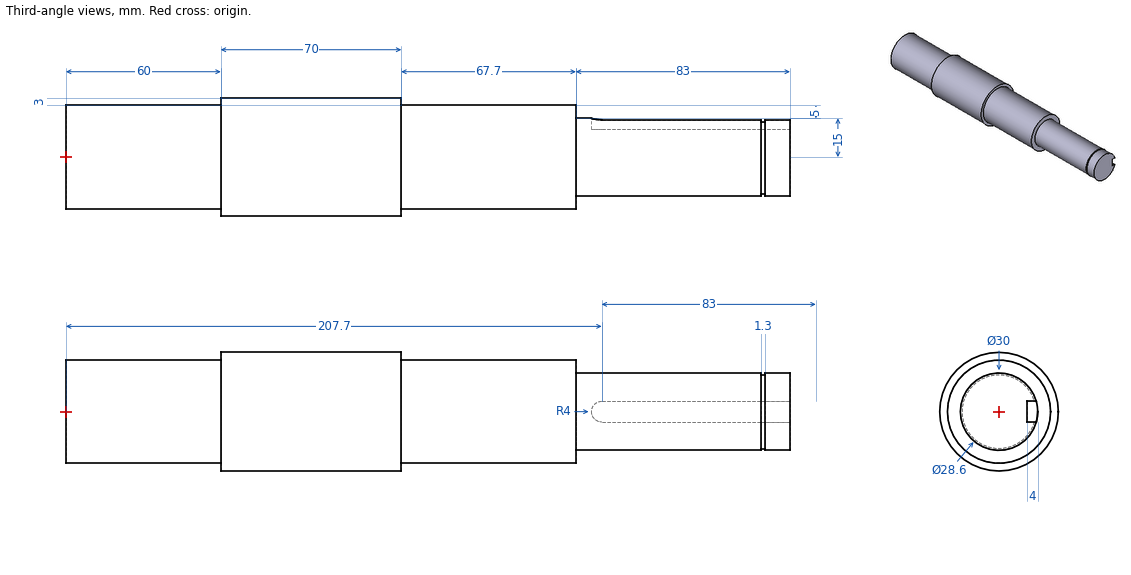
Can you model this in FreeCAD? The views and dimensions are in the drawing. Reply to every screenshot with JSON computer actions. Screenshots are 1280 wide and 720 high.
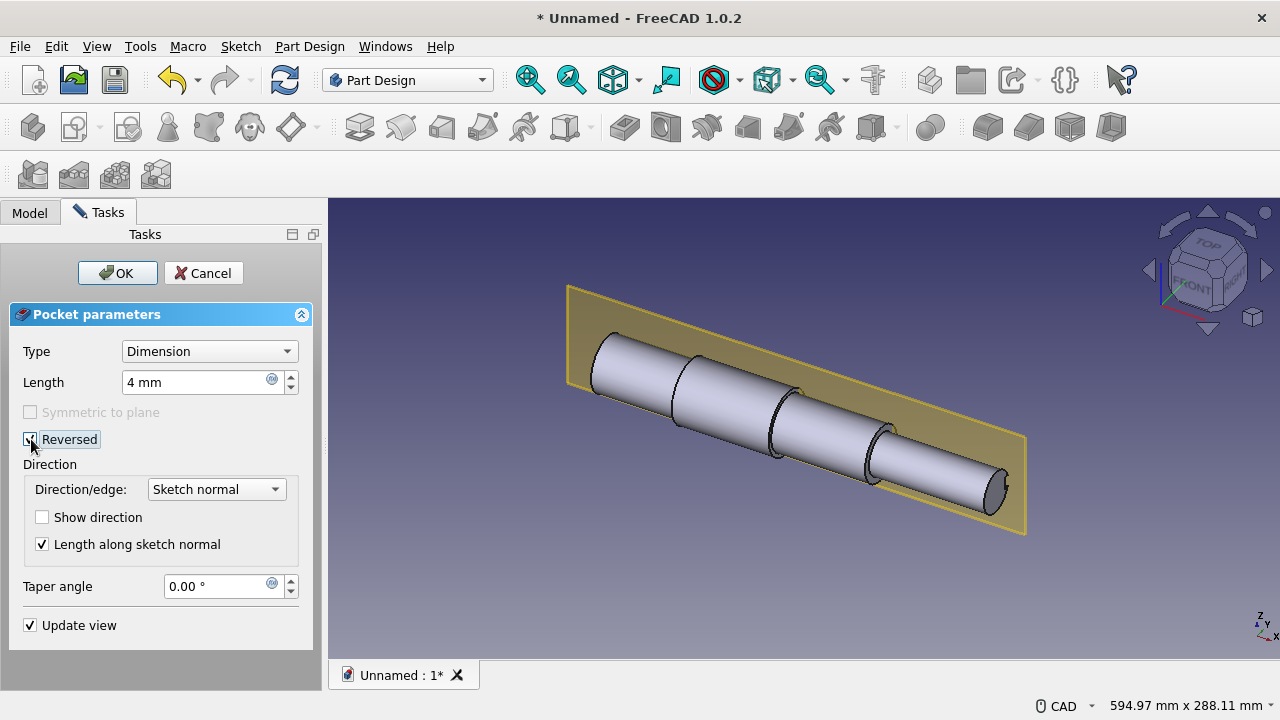
{"action": "left_click", "coordinate": [118, 273]}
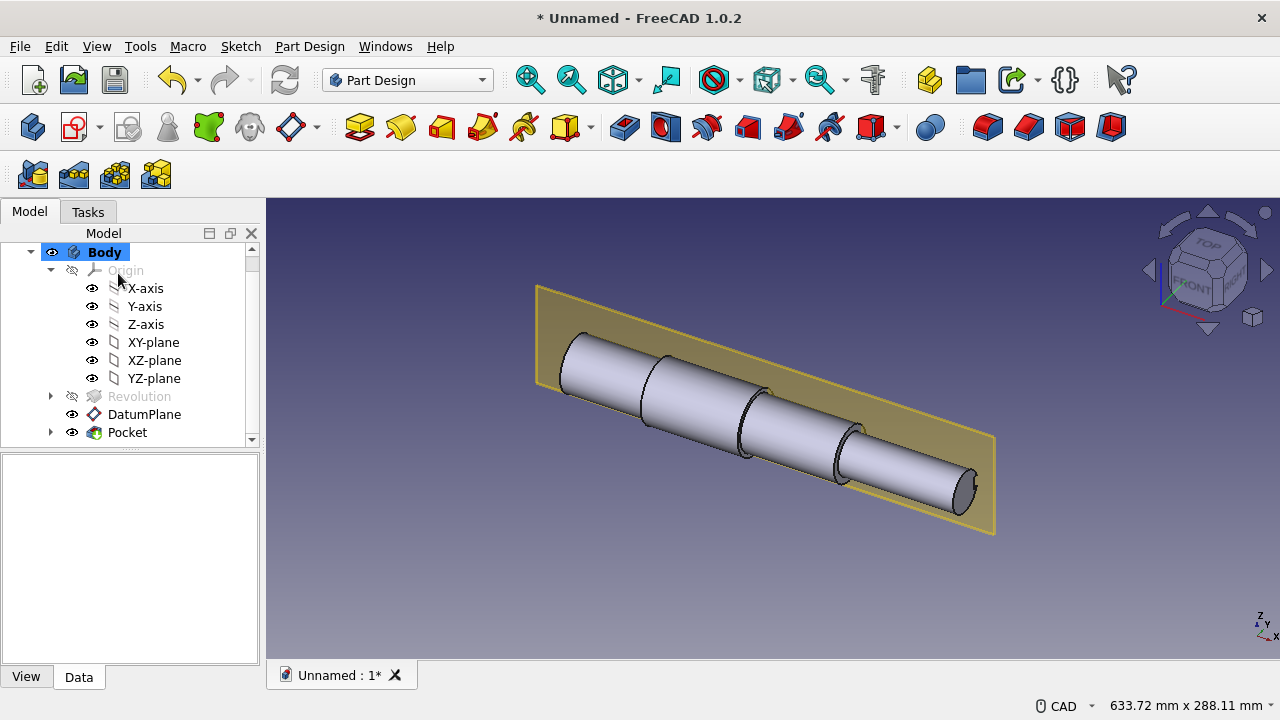
{"action": "left_click", "coordinate": [117, 414]}
{"action": "key", "text": "space"}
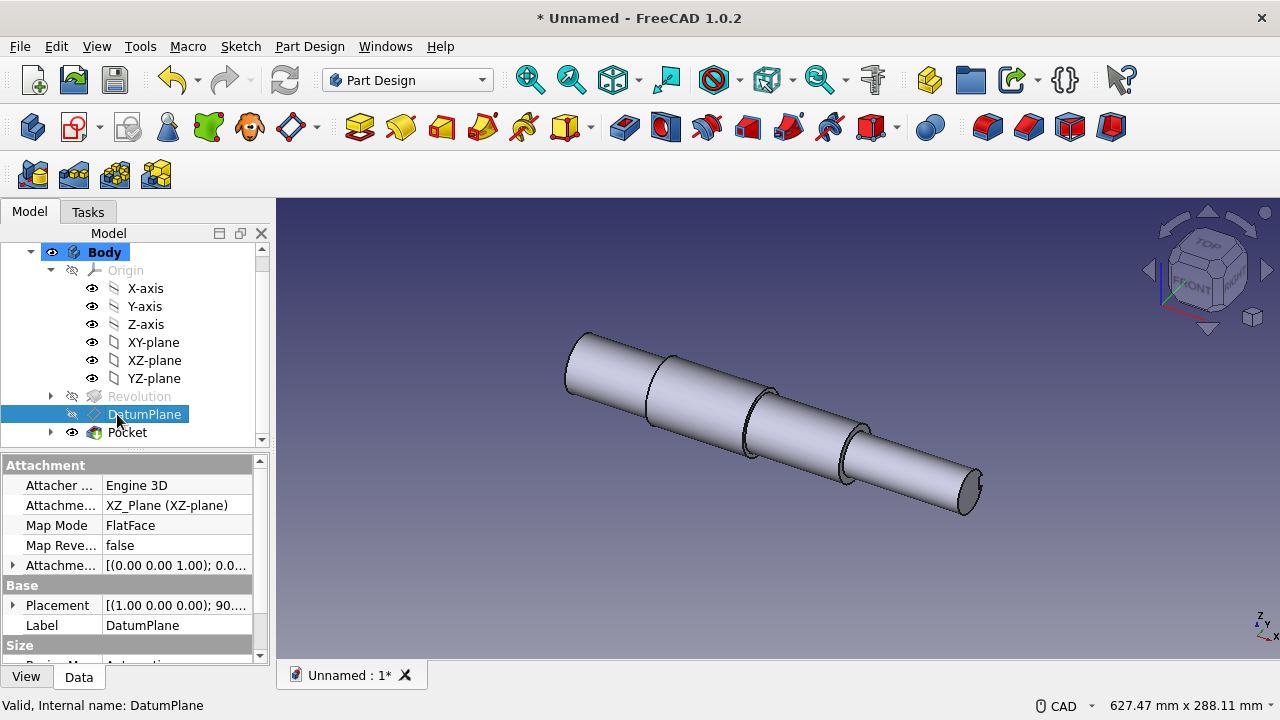
{"action": "left_click", "coordinate": [137, 378]}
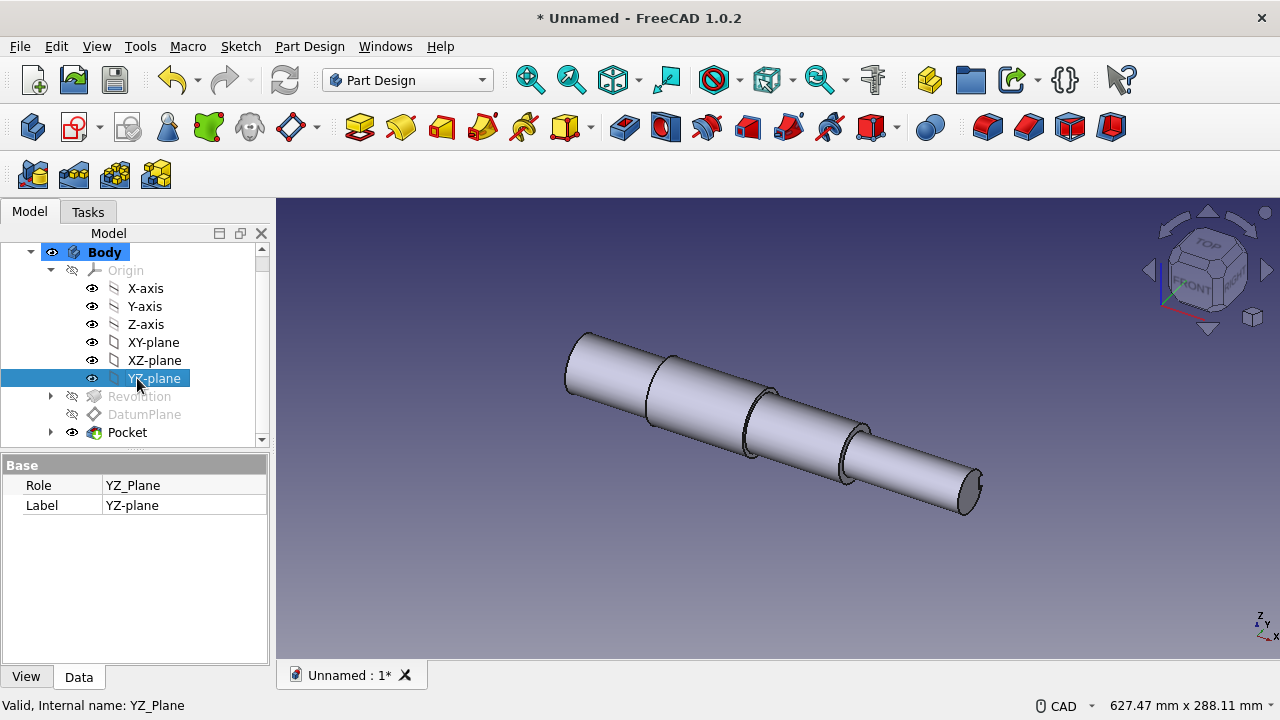
{"action": "left_click", "coordinate": [290, 128]}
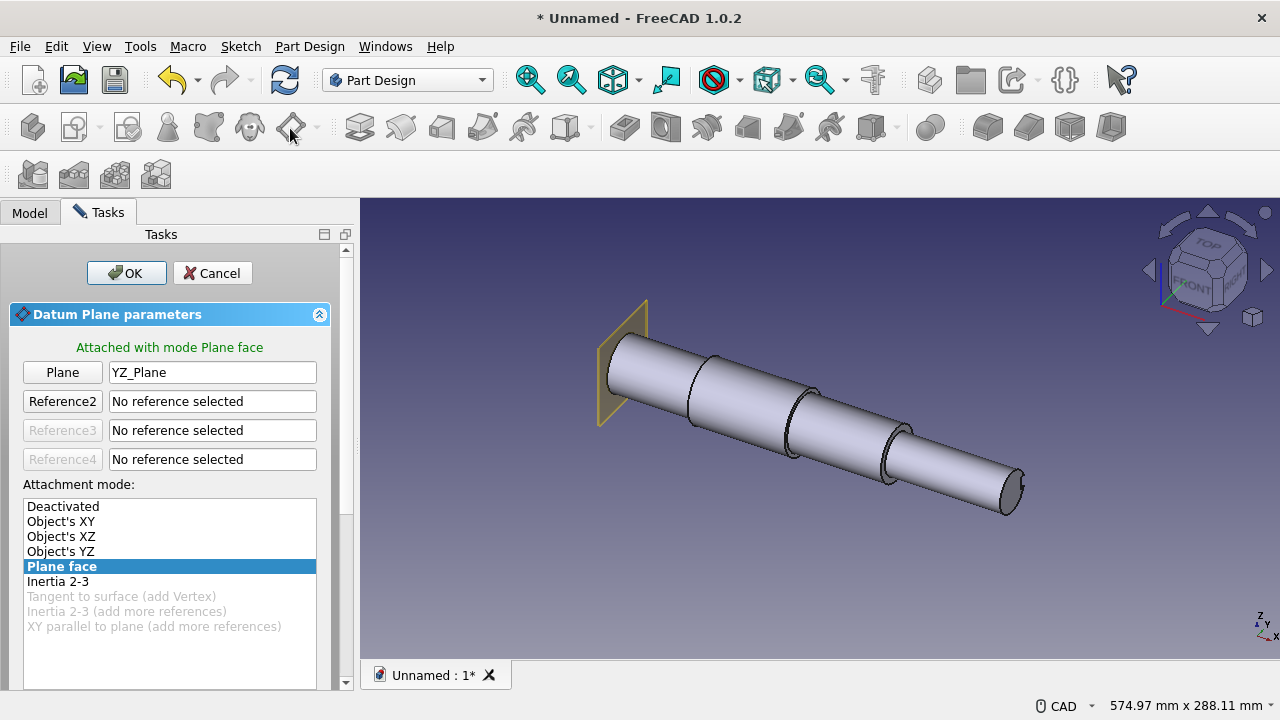
{"action": "scroll", "coordinate": [346, 467], "scroll_direction": "down", "scroll_amount": 4}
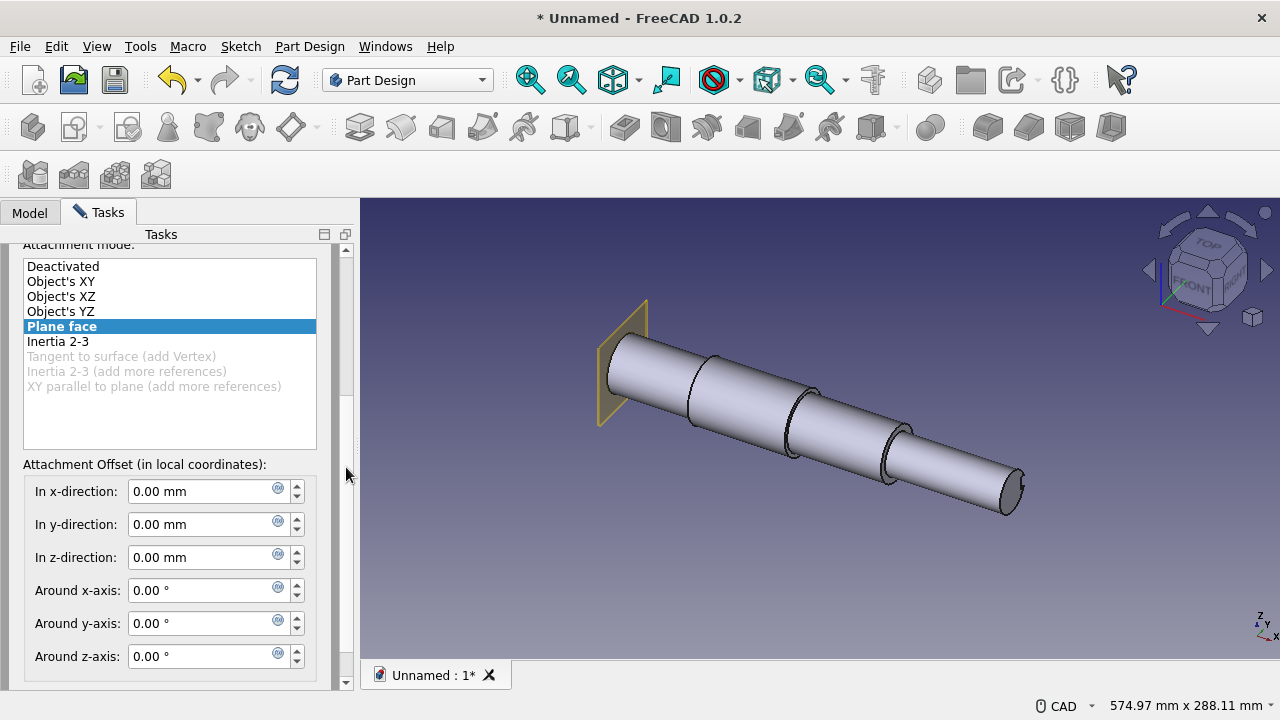
{"action": "triple_click", "coordinate": [210, 558]}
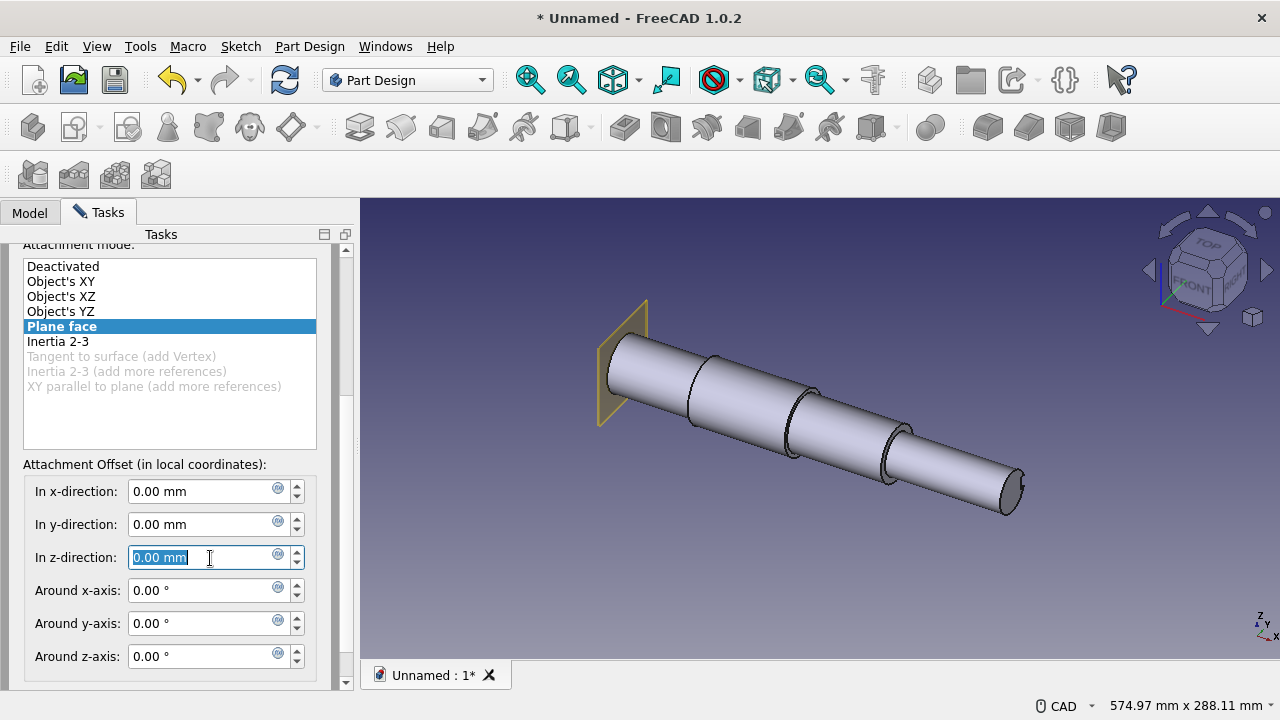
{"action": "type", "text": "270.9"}
{"action": "key", "text": "Tab"}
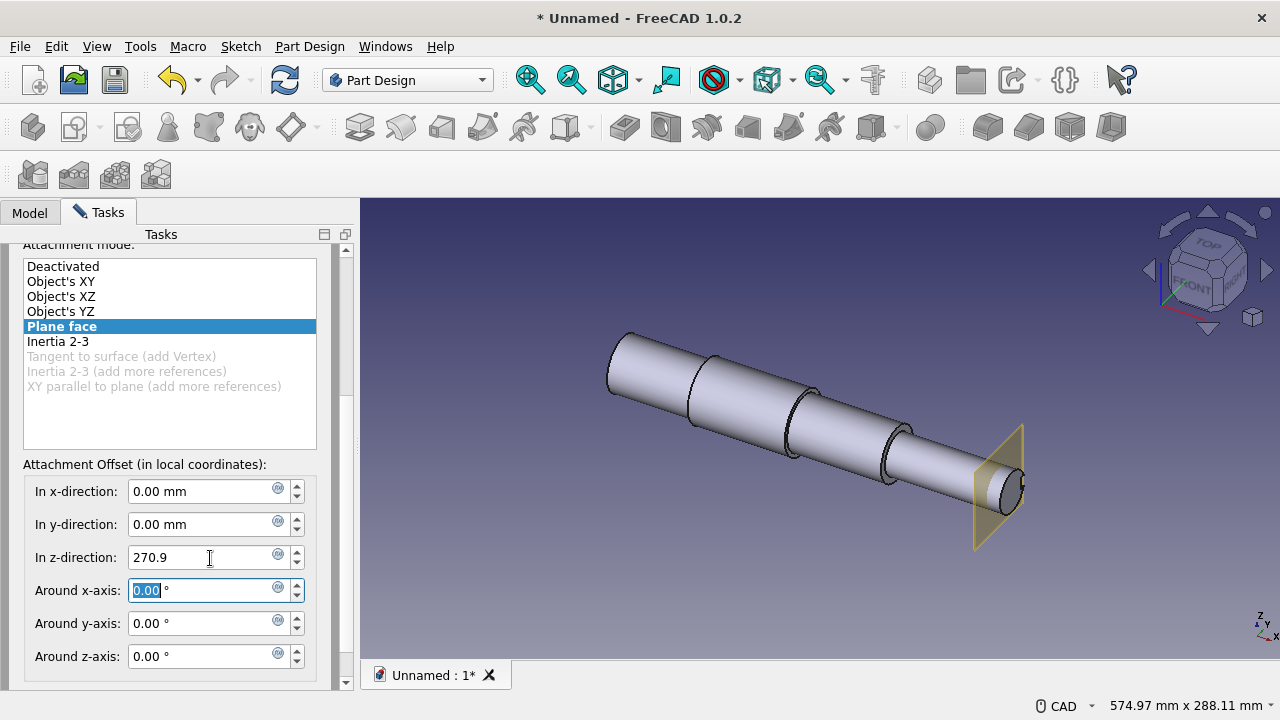
{"action": "scroll", "coordinate": [346, 467], "scroll_direction": "up", "scroll_amount": 5}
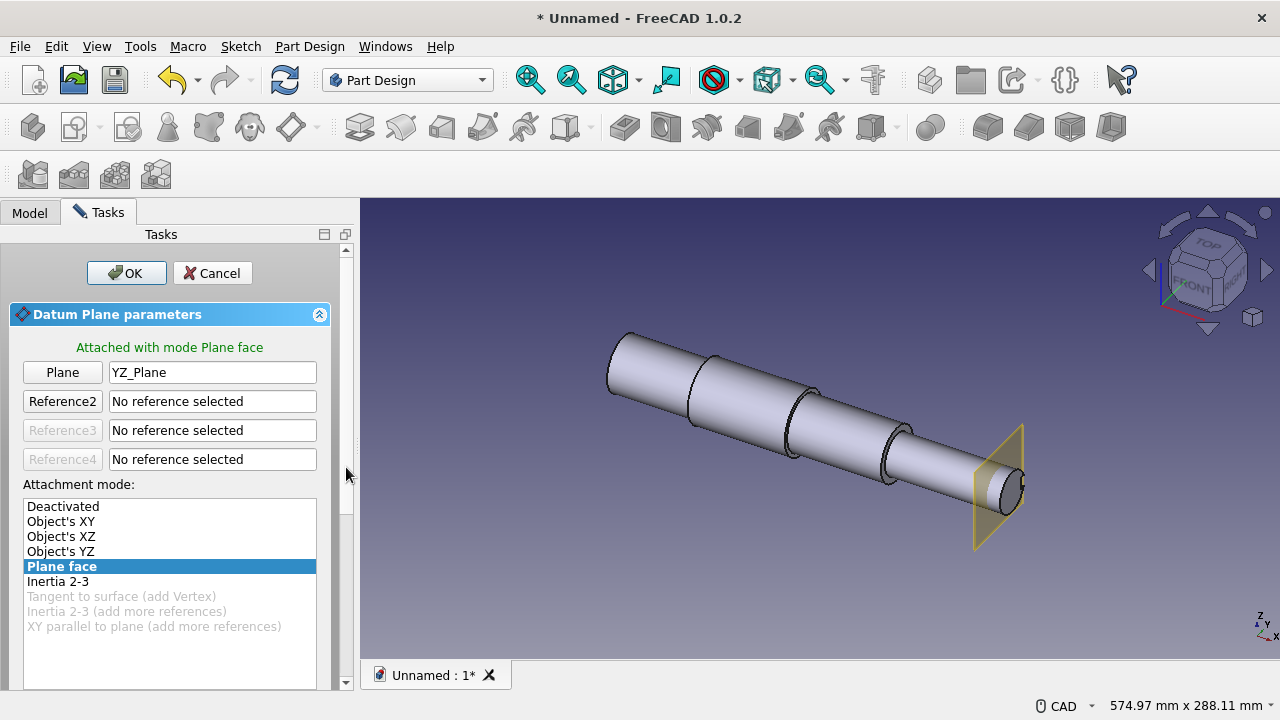
{"action": "left_click", "coordinate": [127, 273]}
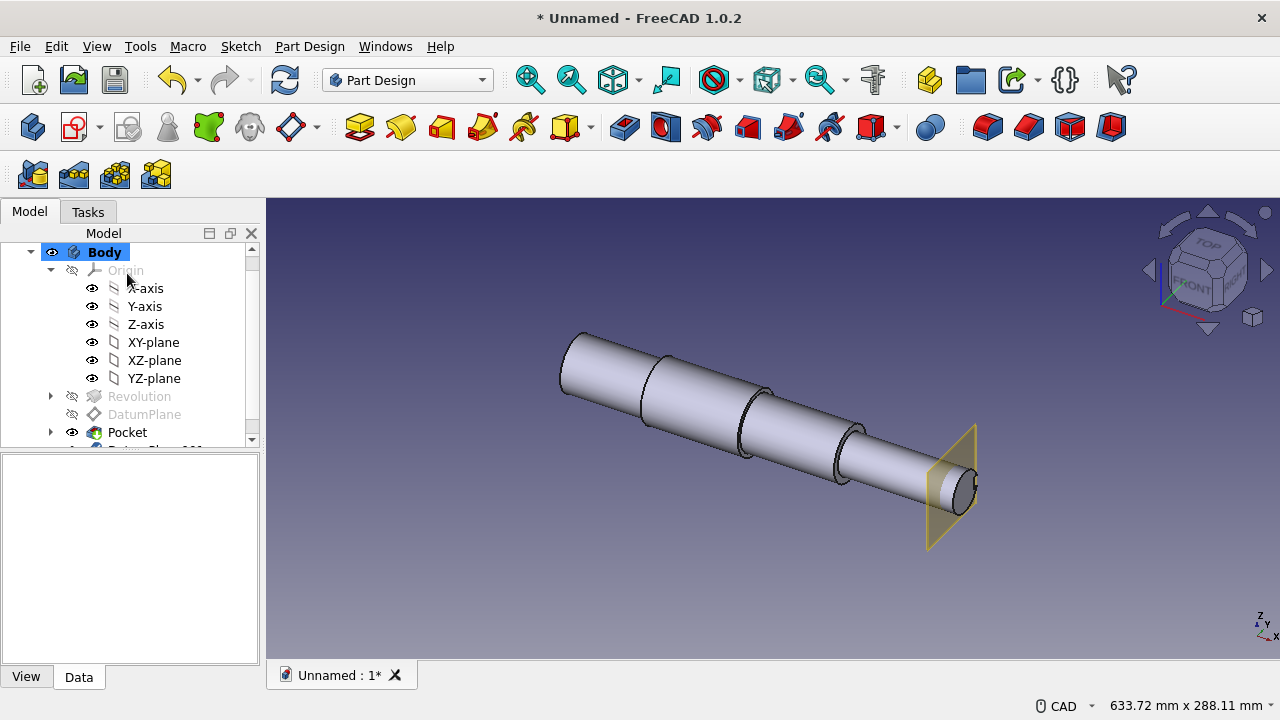
{"action": "scroll", "coordinate": [121, 338], "scroll_direction": "down", "scroll_amount": 3}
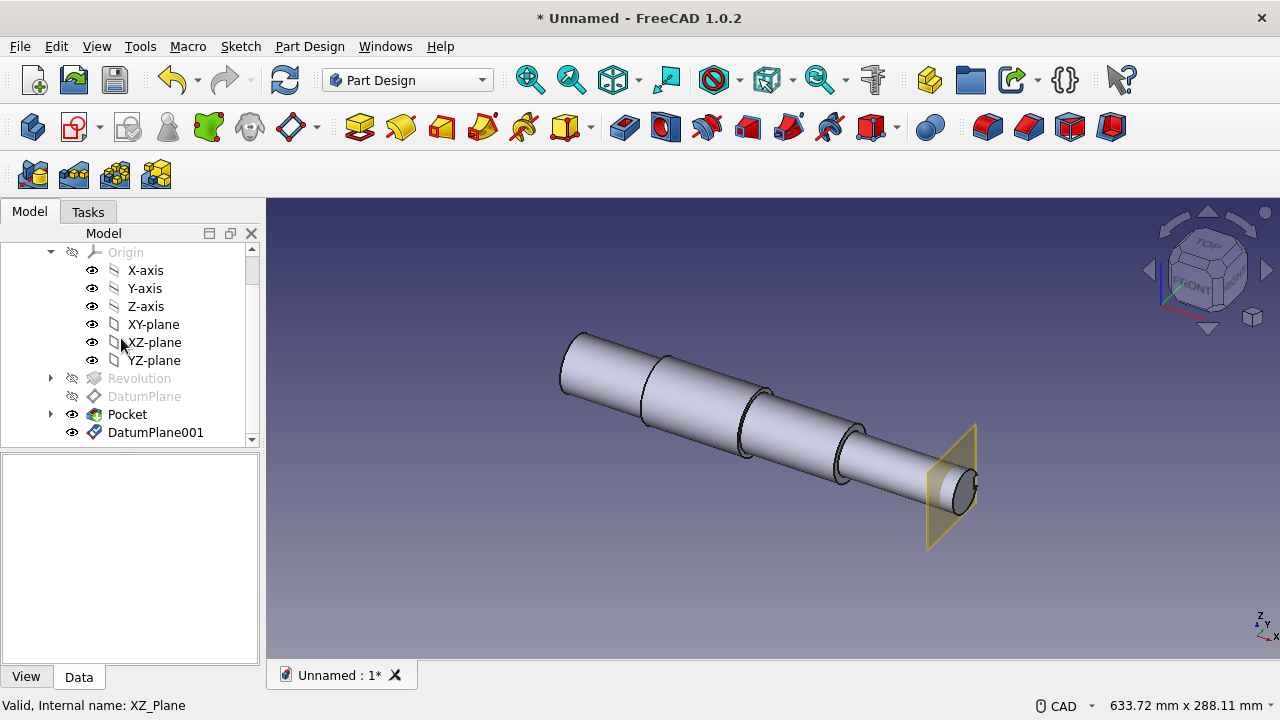
{"action": "left_click", "coordinate": [117, 432]}